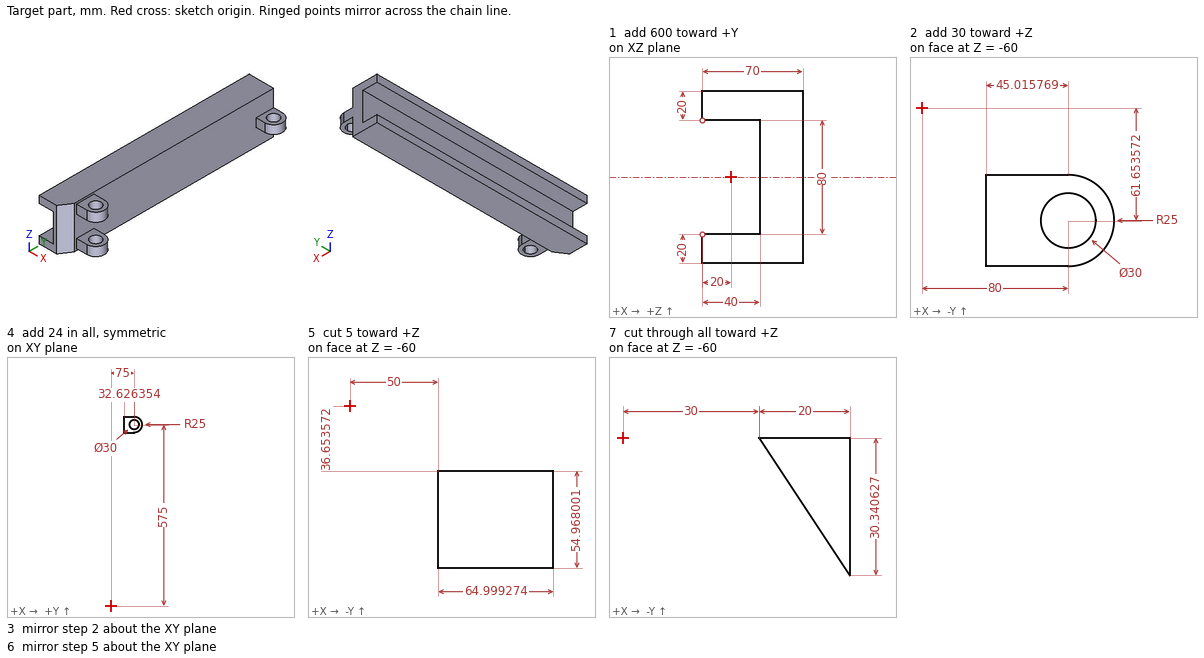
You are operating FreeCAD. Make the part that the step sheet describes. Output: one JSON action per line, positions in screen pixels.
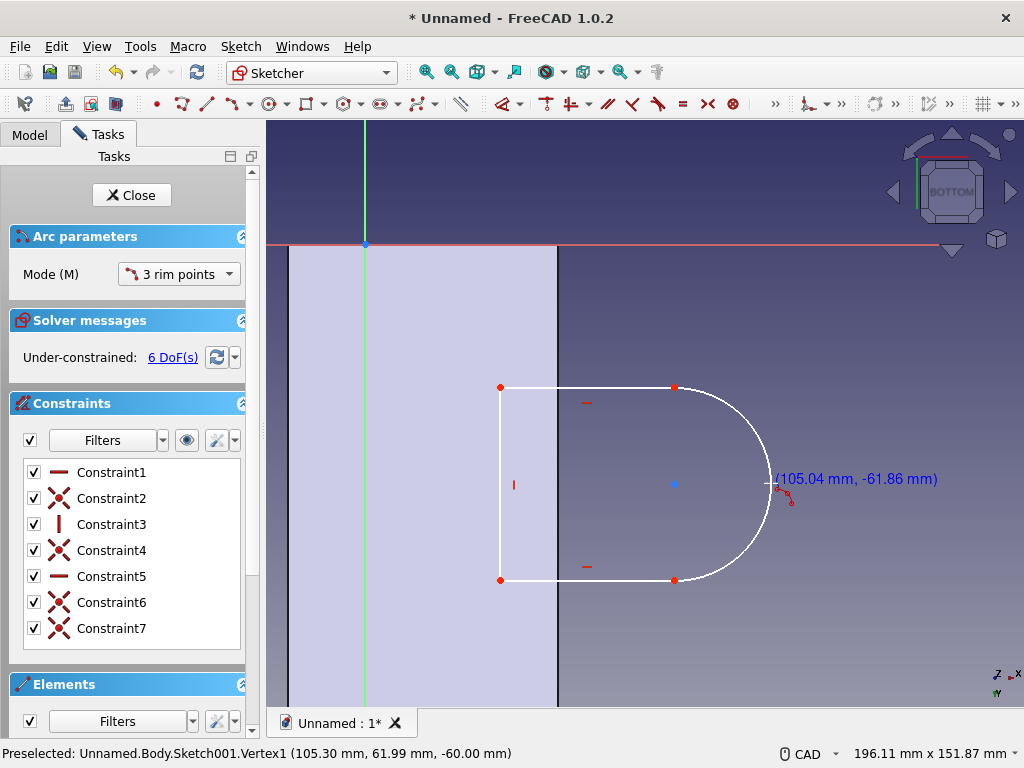
{"action": "left_click", "coordinate": [268, 104]}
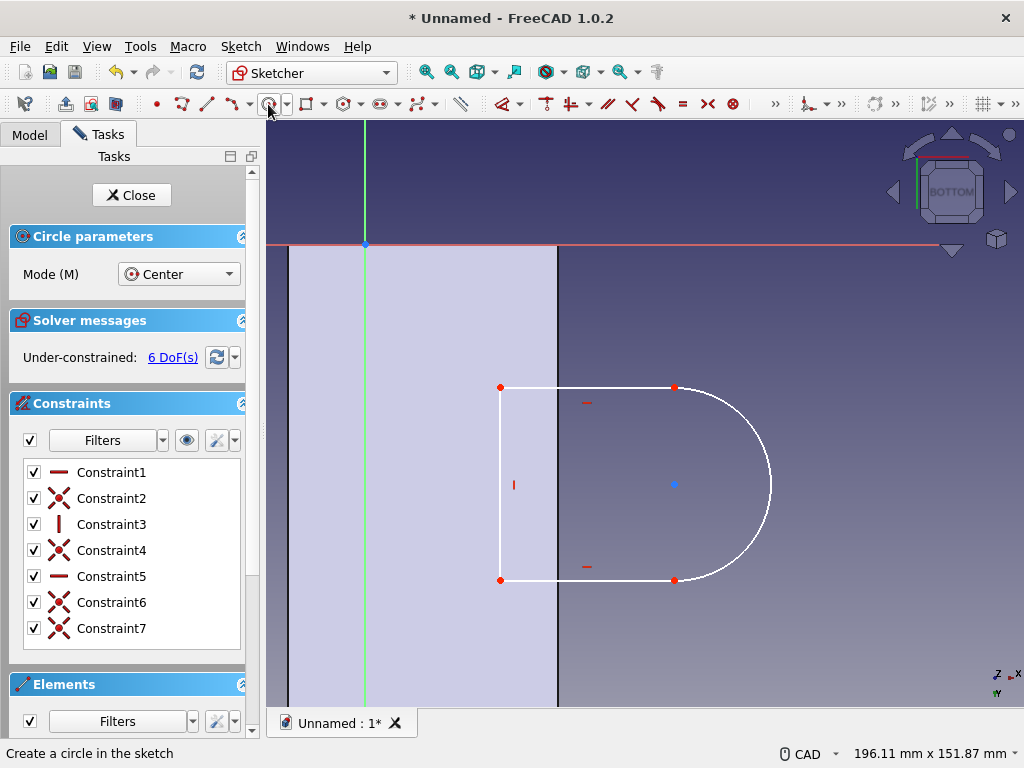
{"action": "left_click", "coordinate": [674, 483]}
{"action": "mouse_move", "coordinate": [715, 442]}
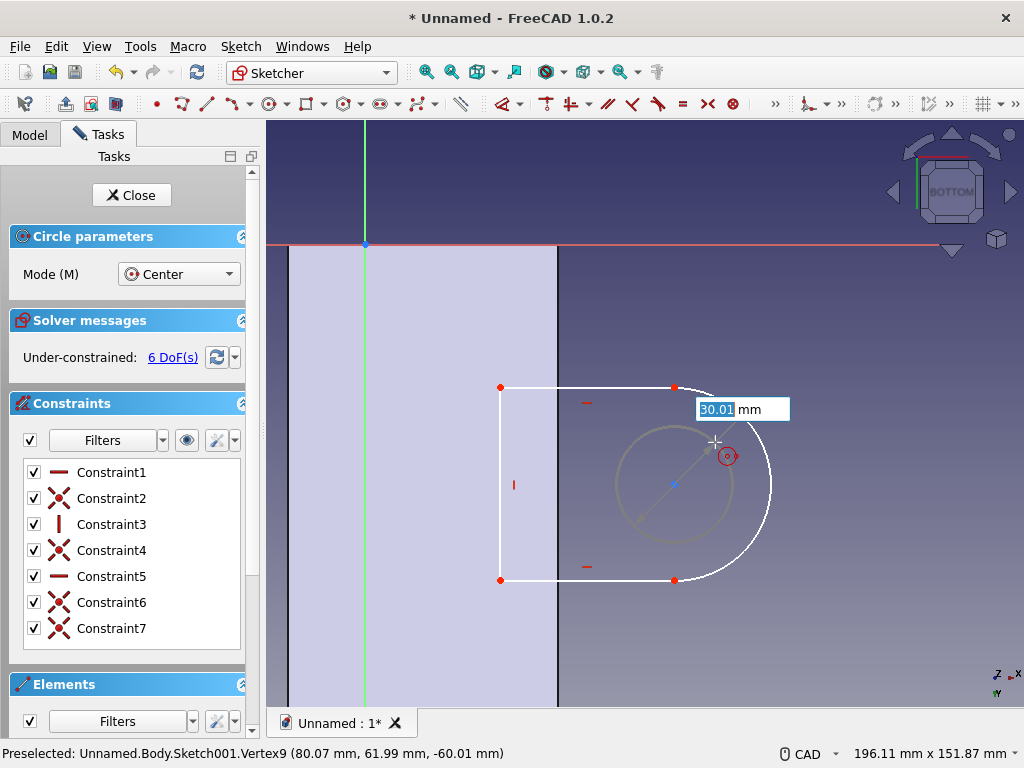
{"action": "type", "text": "30"}
{"action": "key", "text": "Return"}
{"action": "key", "text": "Escape"}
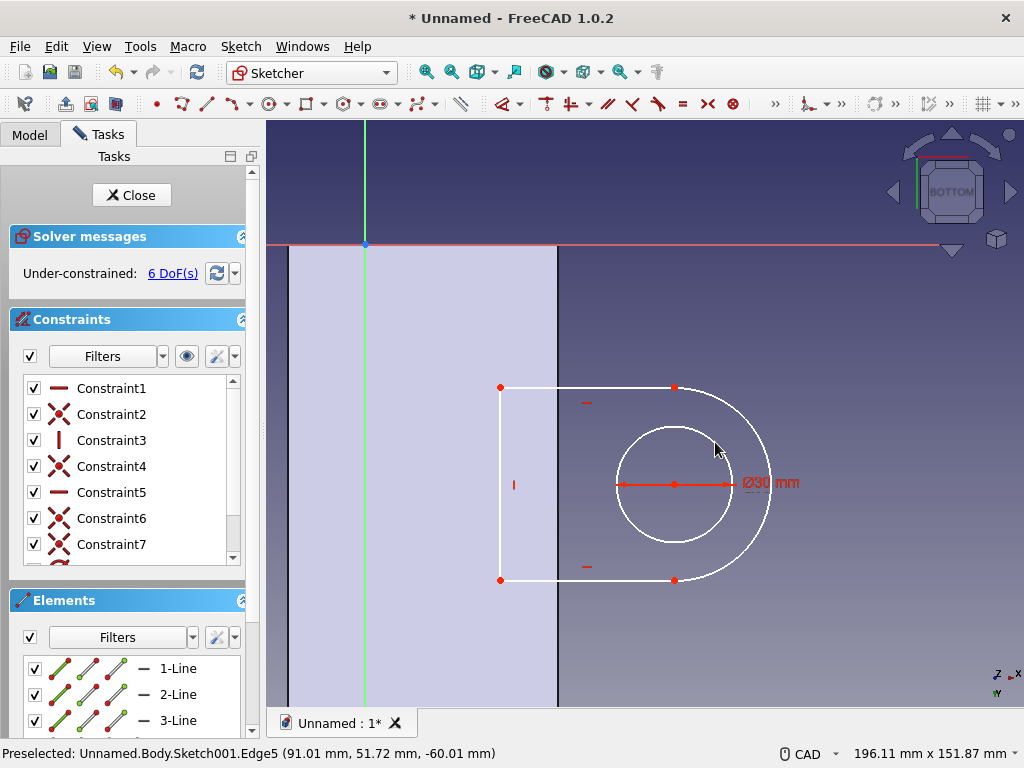
{"action": "left_click", "coordinate": [622, 388]}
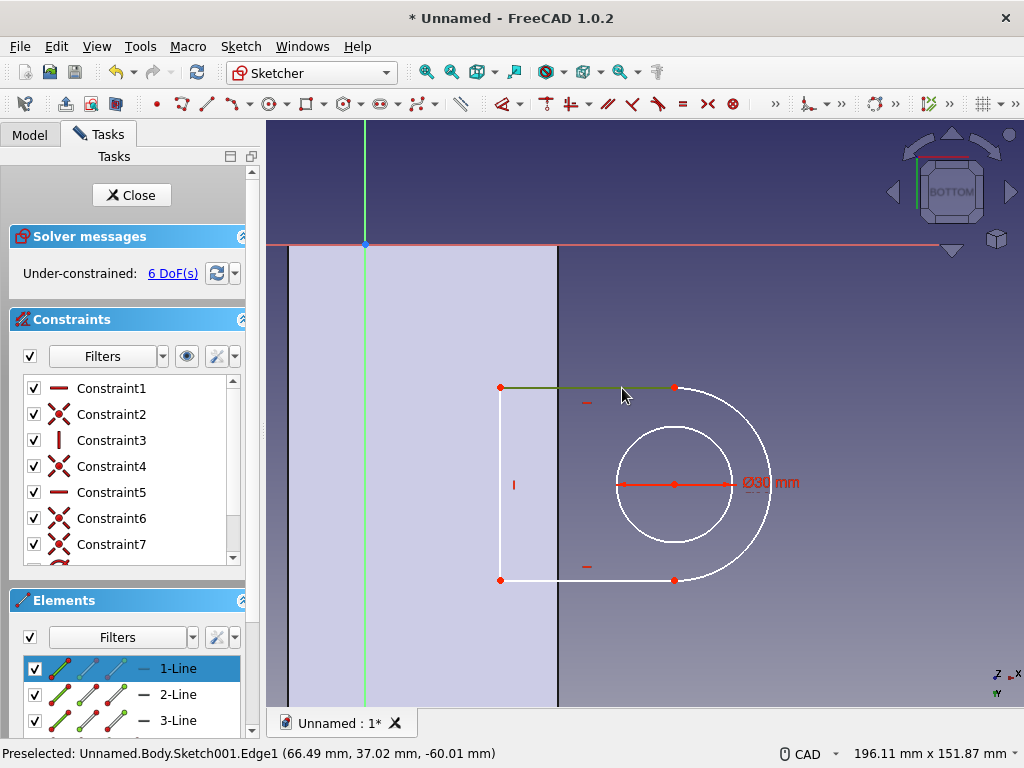
{"action": "left_click", "coordinate": [752, 541]}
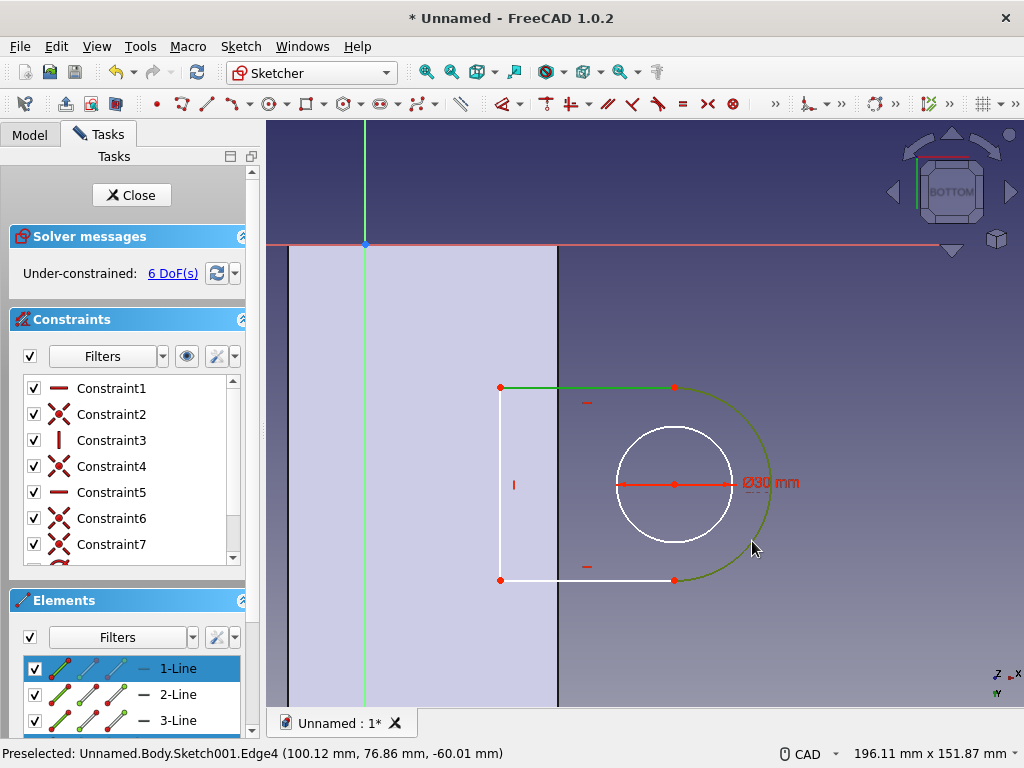
{"action": "left_click", "coordinate": [658, 104]}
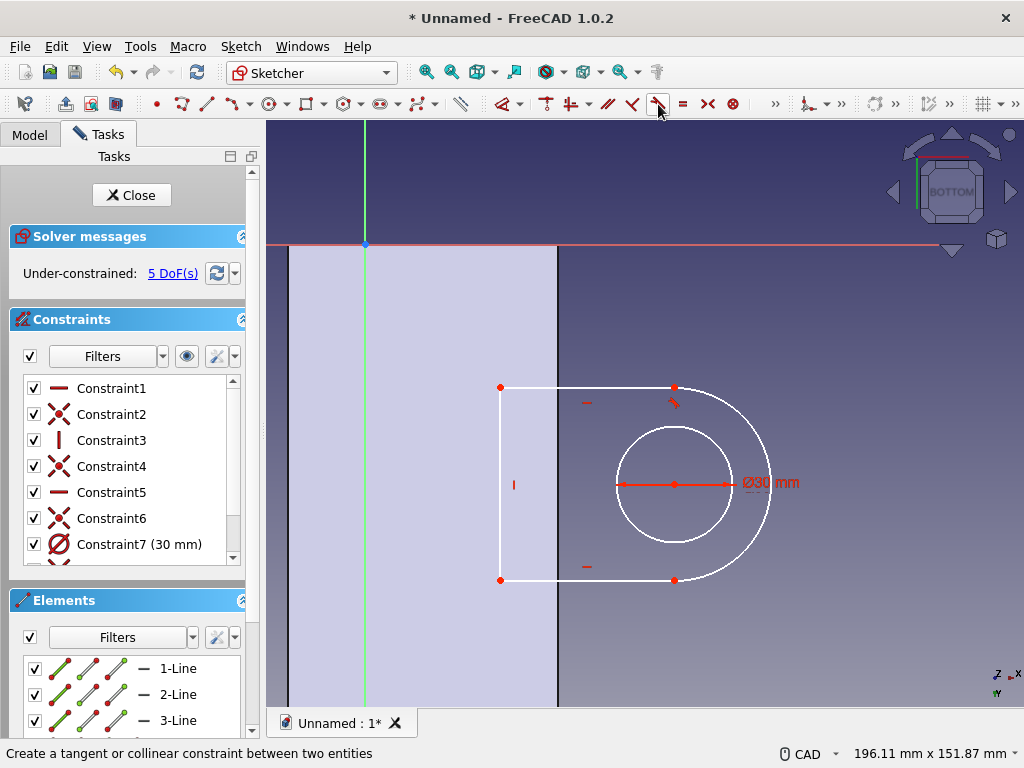
{"action": "left_click", "coordinate": [552, 581]}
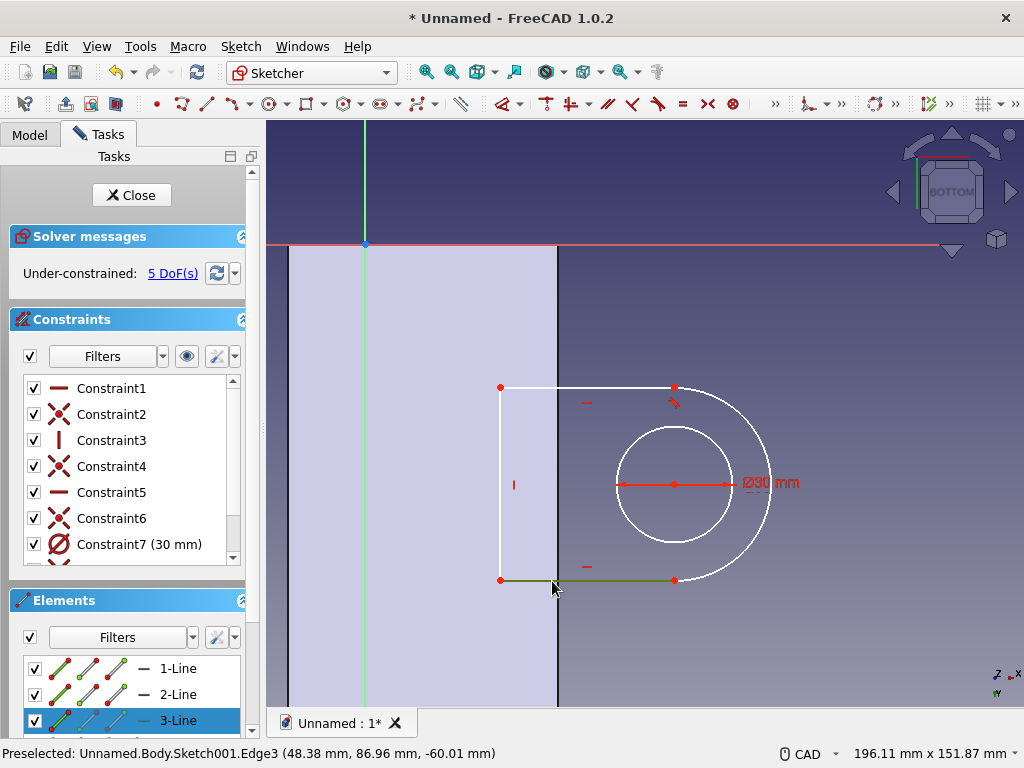
{"action": "left_click", "coordinate": [752, 542]}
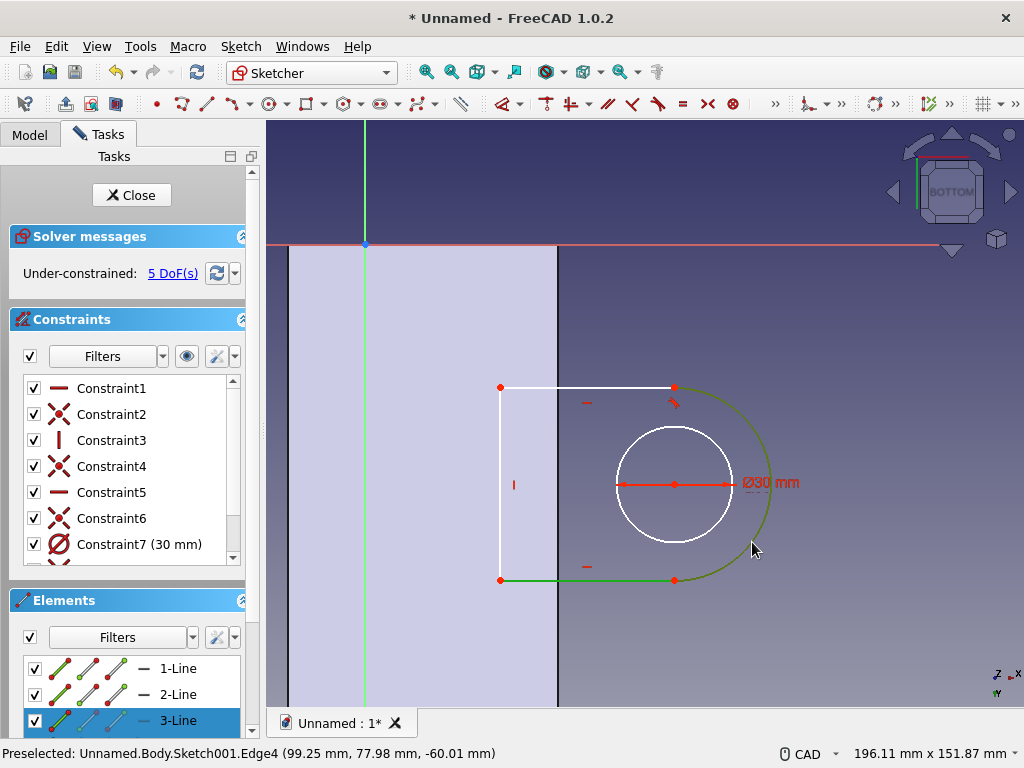
{"action": "left_click", "coordinate": [658, 104]}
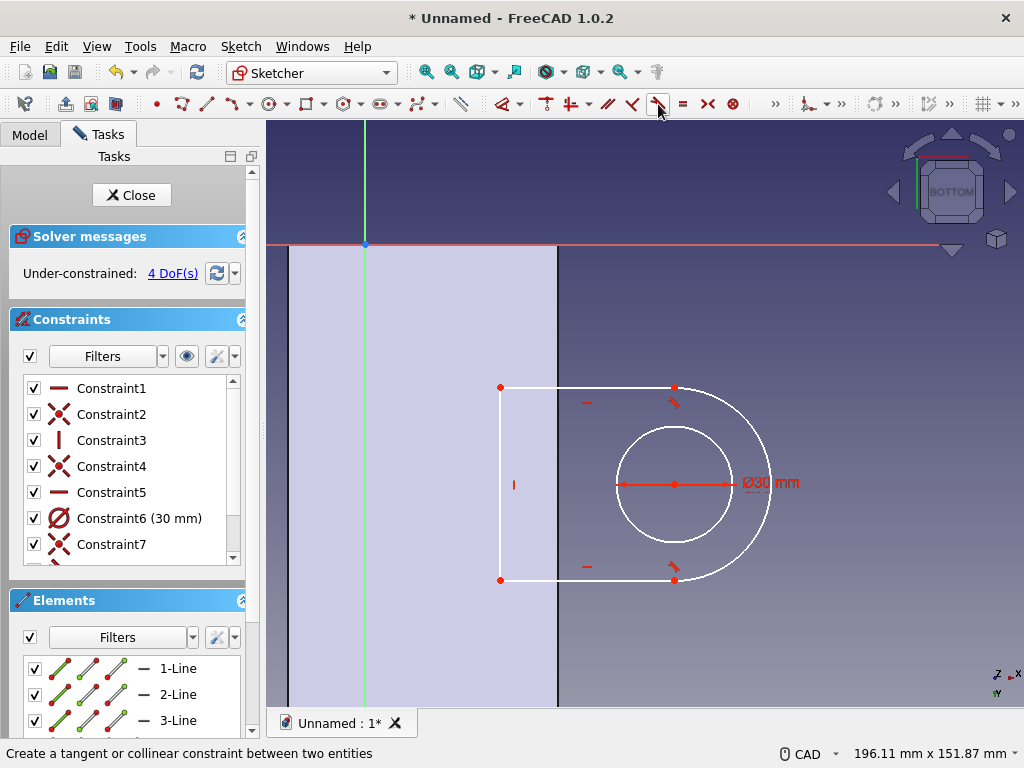
{"action": "left_click", "coordinate": [502, 104]}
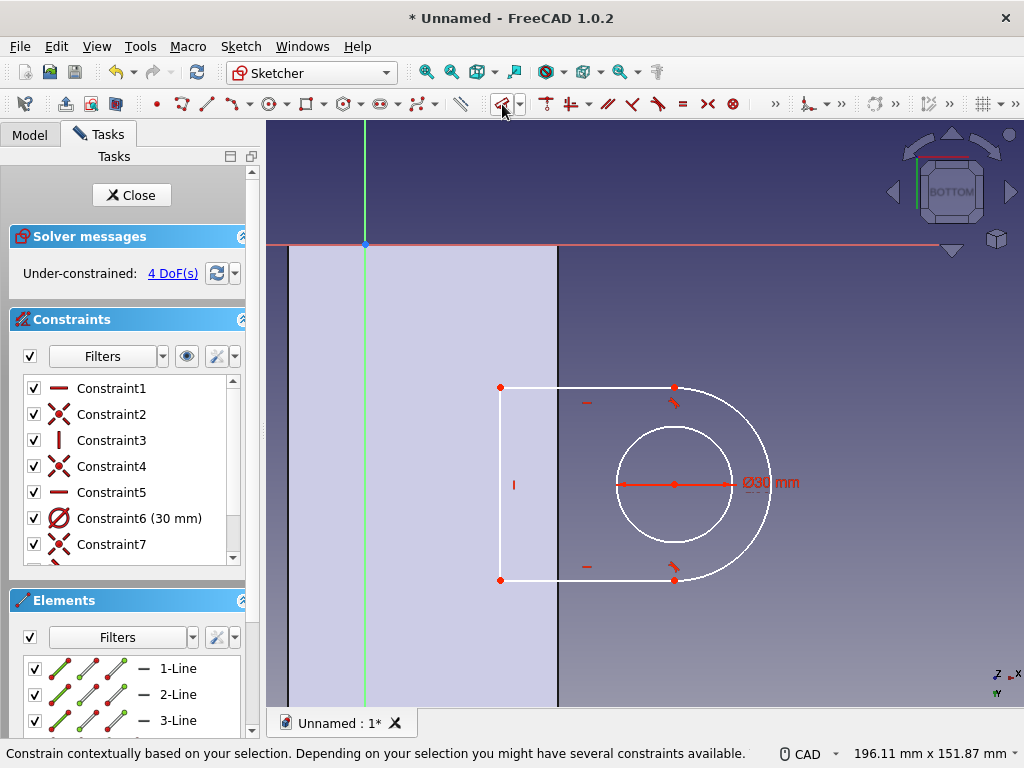
{"action": "left_click", "coordinate": [753, 541]}
{"action": "left_click", "coordinate": [779, 560]}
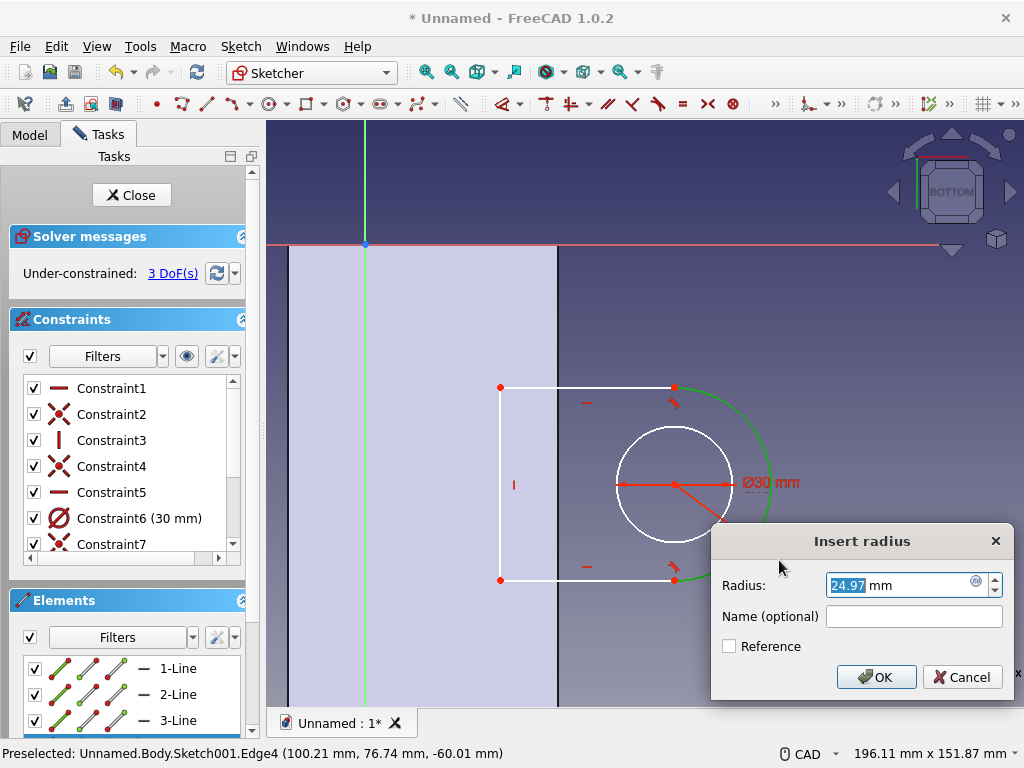
{"action": "type", "text": "25"}
{"action": "key", "text": "Return"}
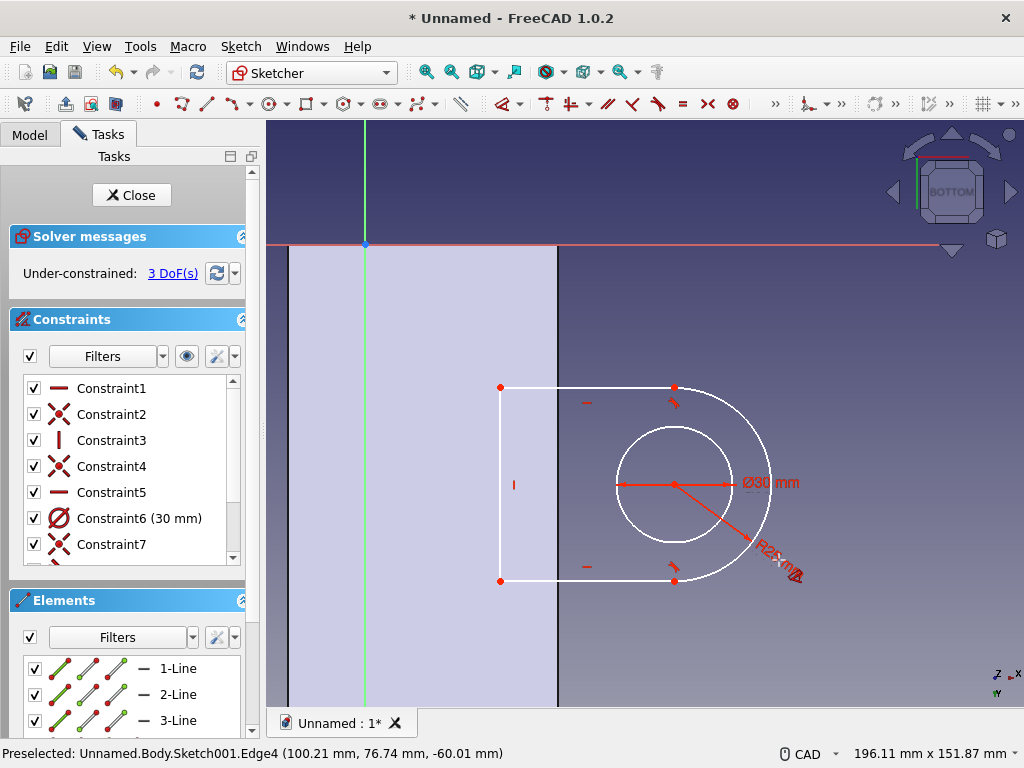
{"action": "left_click", "coordinate": [674, 485]}
{"action": "left_click", "coordinate": [520, 211]}